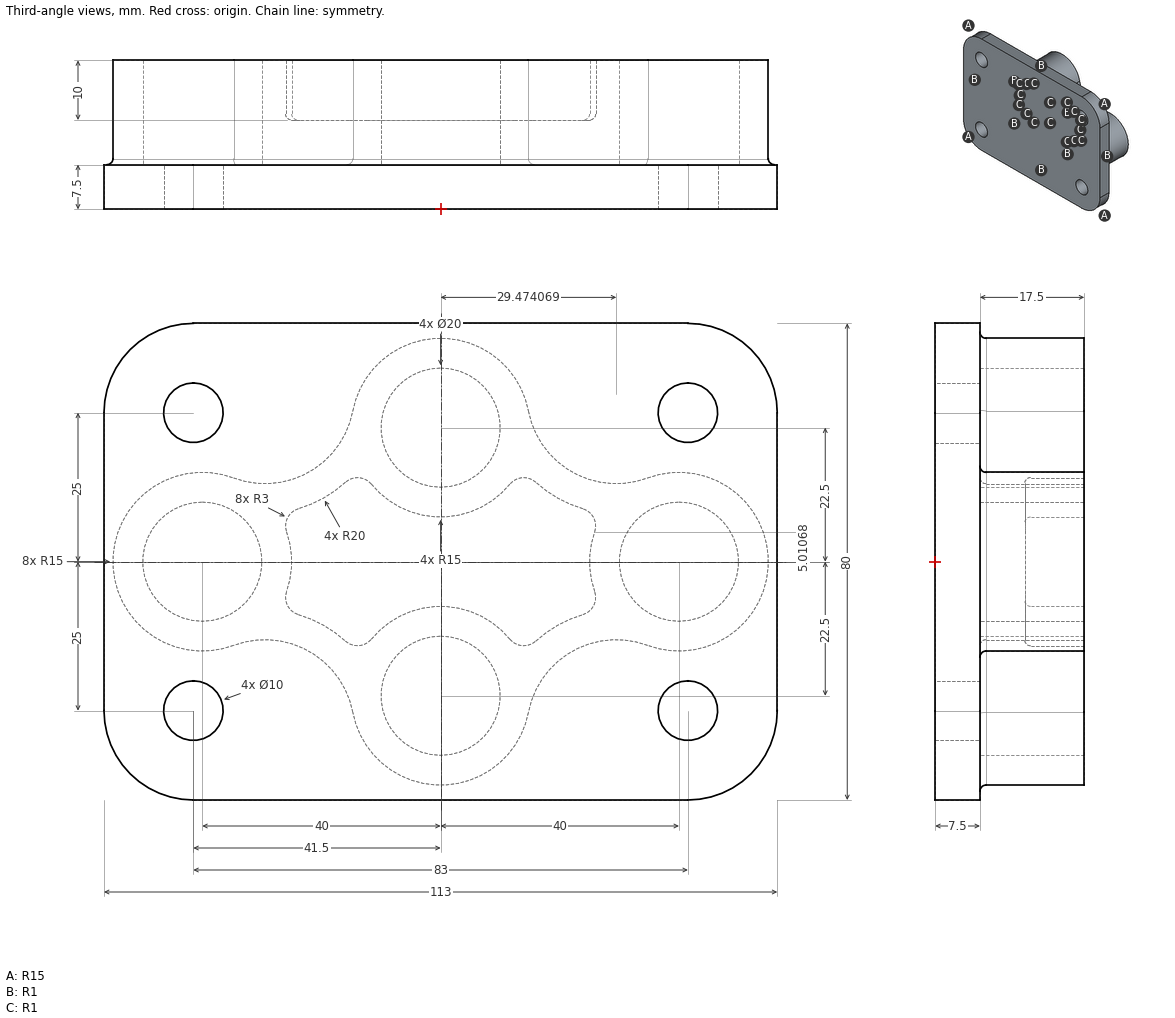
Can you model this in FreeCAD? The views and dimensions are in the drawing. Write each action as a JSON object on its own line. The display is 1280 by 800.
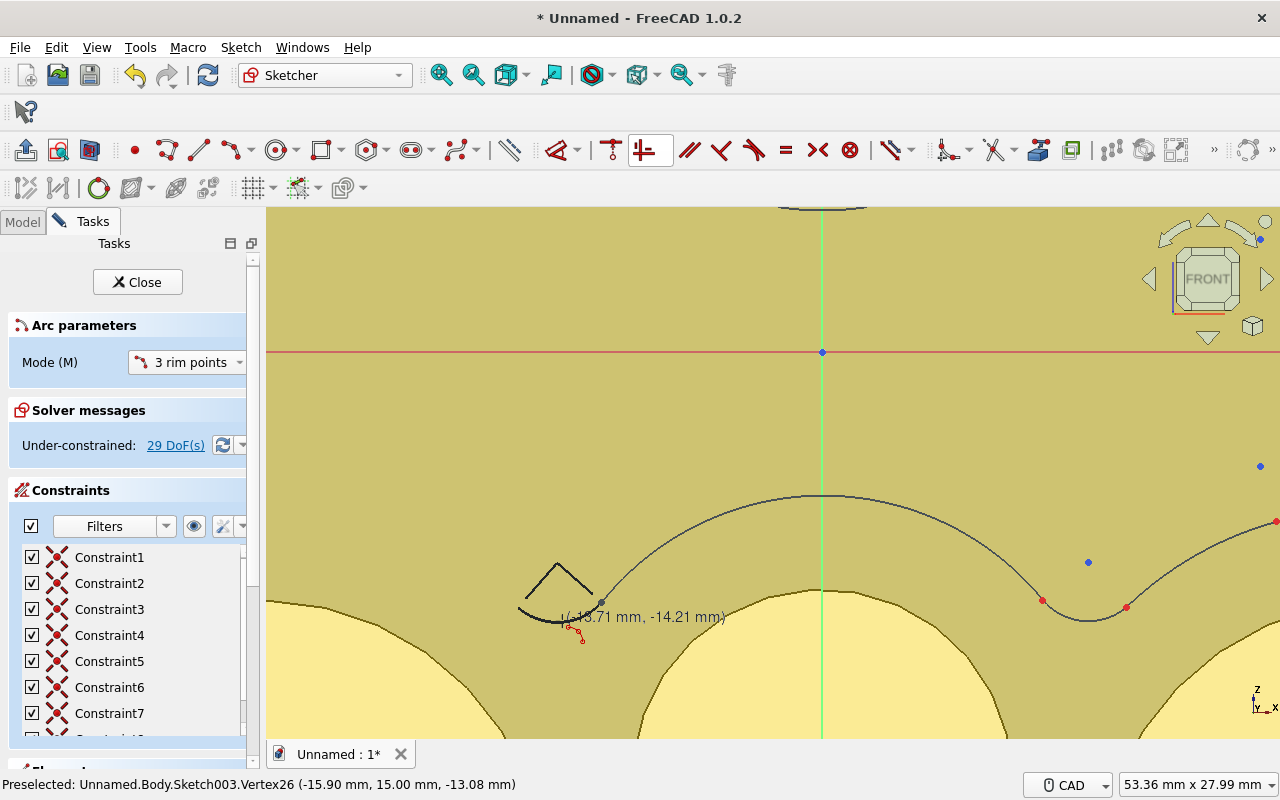
{"action": "left_click", "coordinate": [561, 620]}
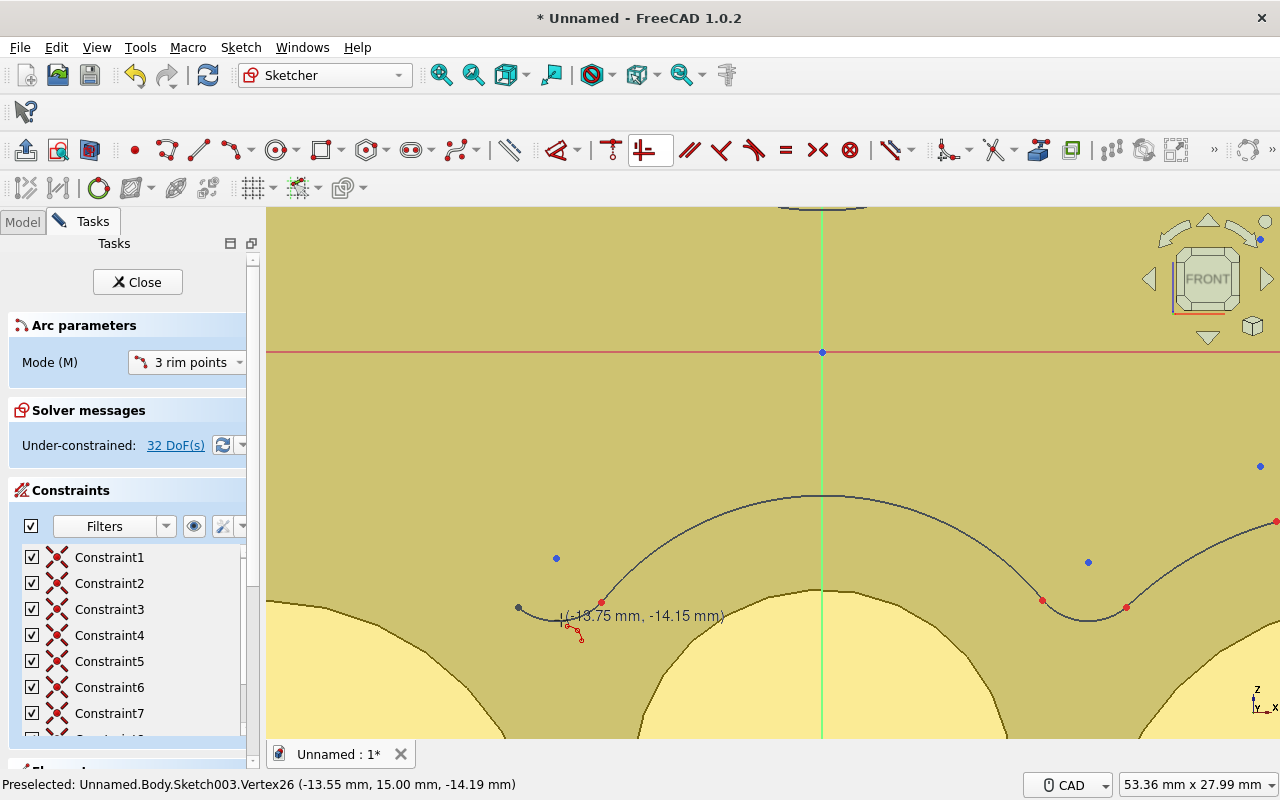
{"action": "left_click", "coordinate": [518, 608]}
{"action": "left_click", "coordinate": [369, 521]}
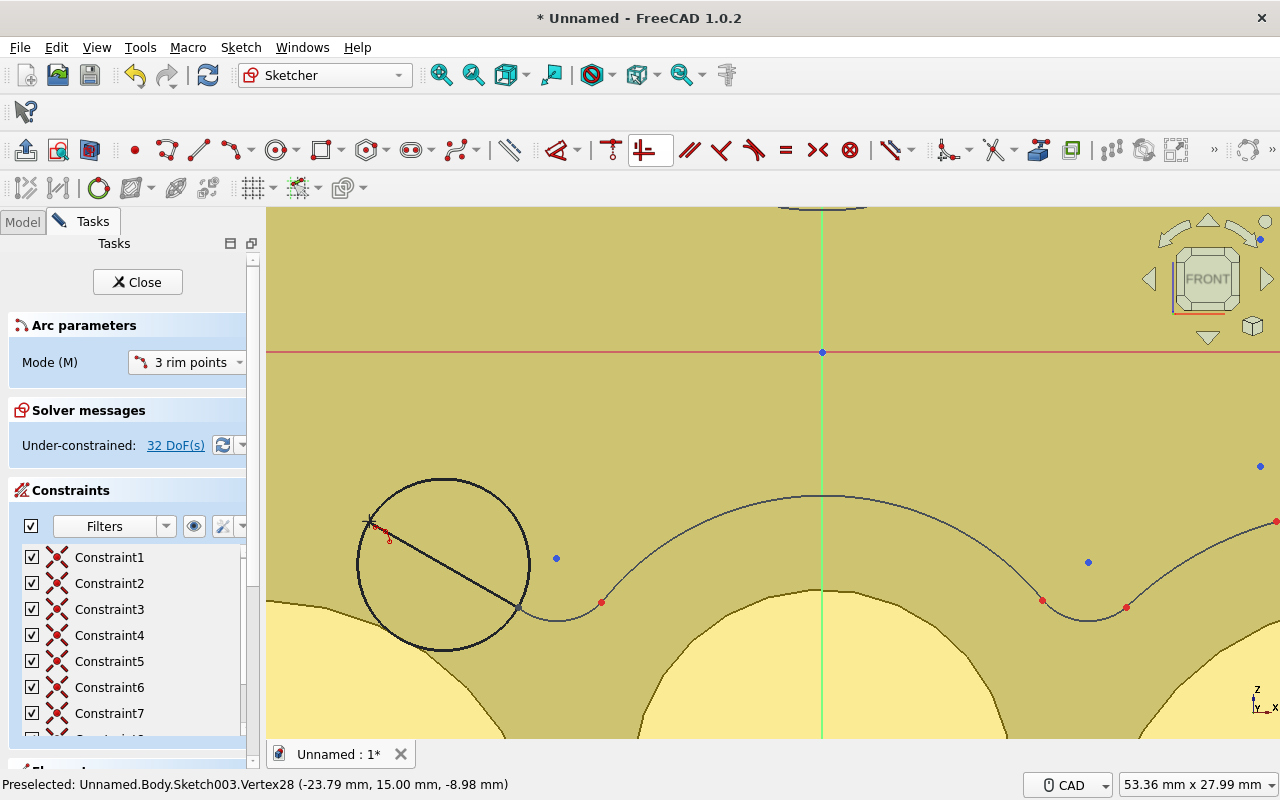
{"action": "scroll", "coordinate": [448, 555], "scroll_direction": "up", "scroll_amount": 3}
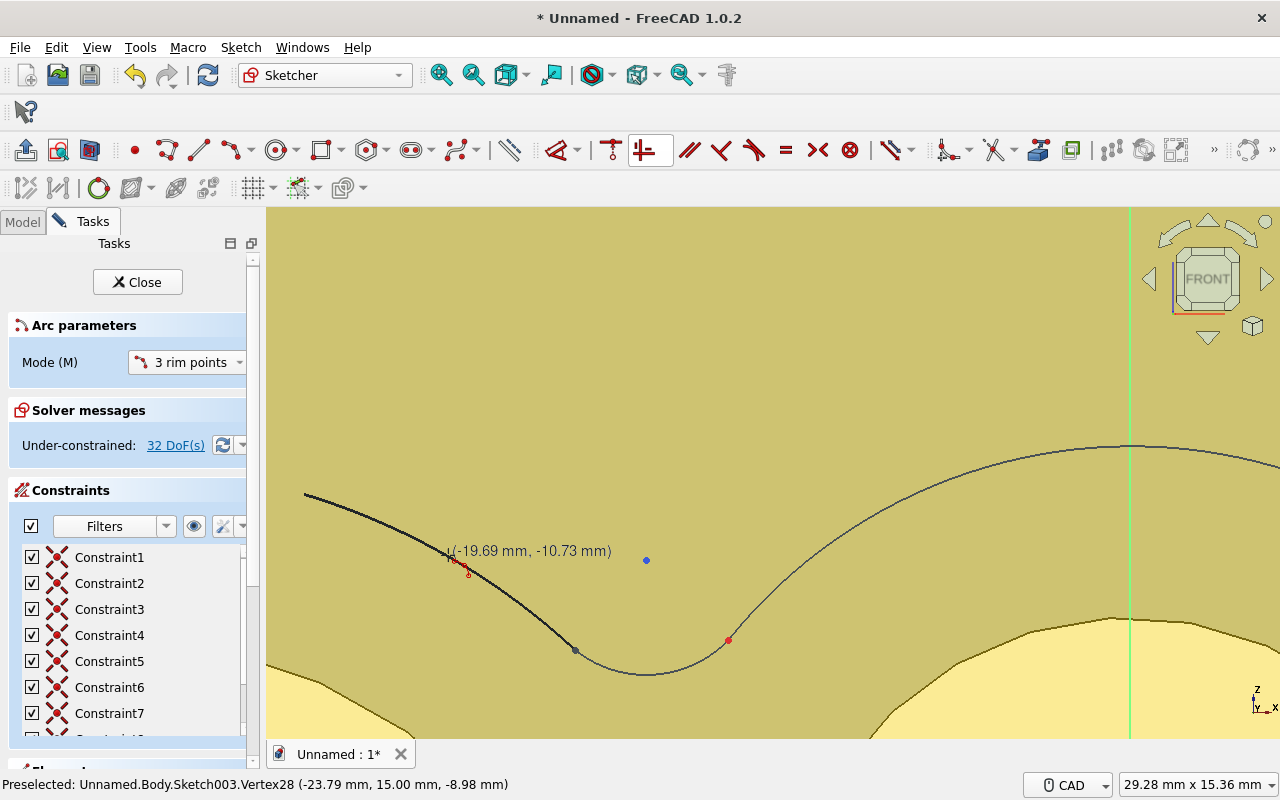
{"action": "left_click", "coordinate": [449, 554]}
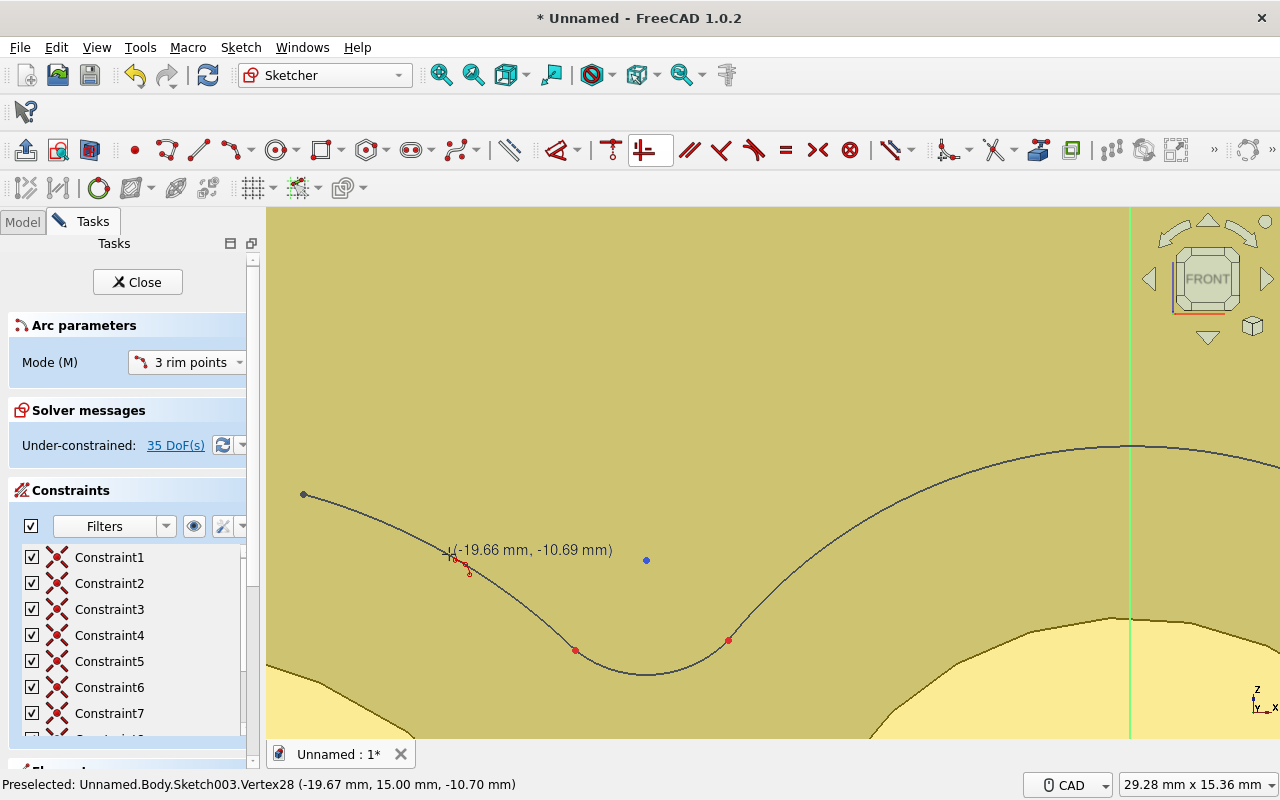
{"action": "left_click", "coordinate": [304, 494]}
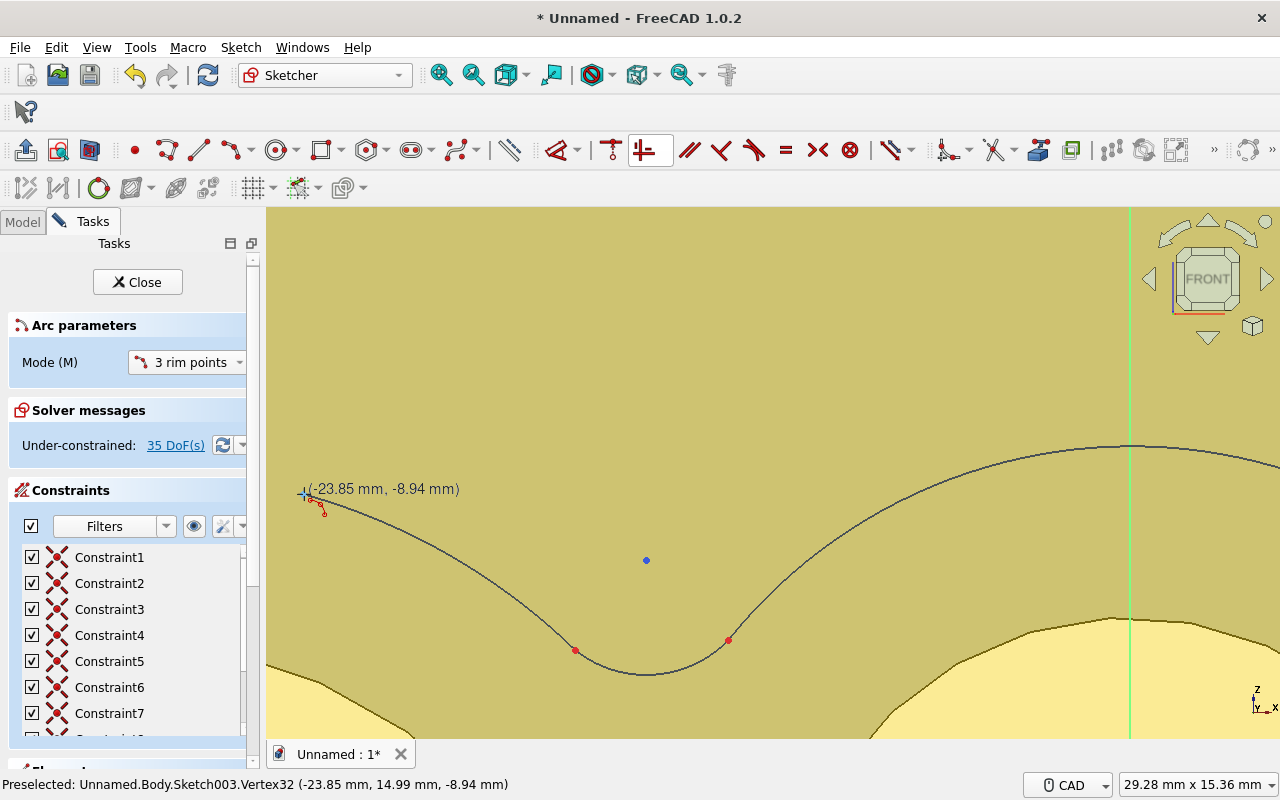
{"action": "scroll", "coordinate": [521, 597], "scroll_direction": "down", "scroll_amount": 6}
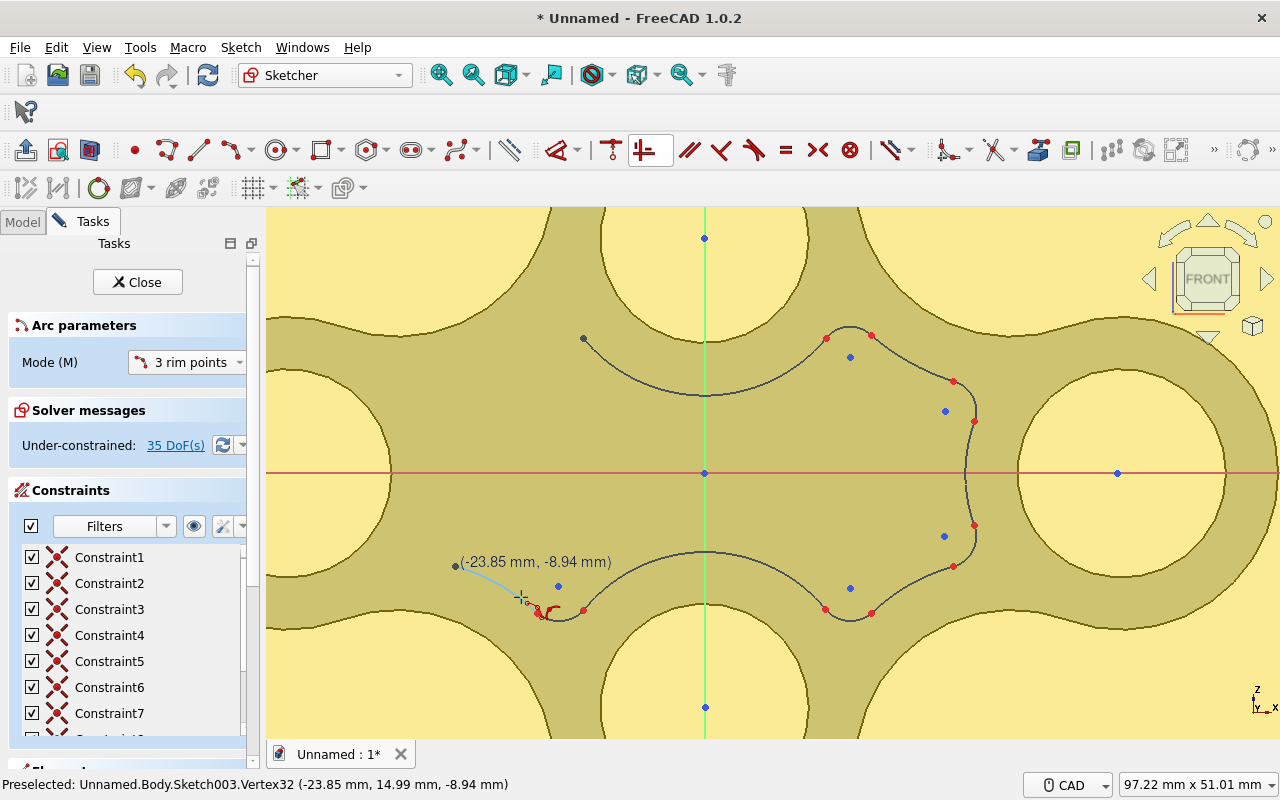
{"action": "left_click", "coordinate": [435, 526]}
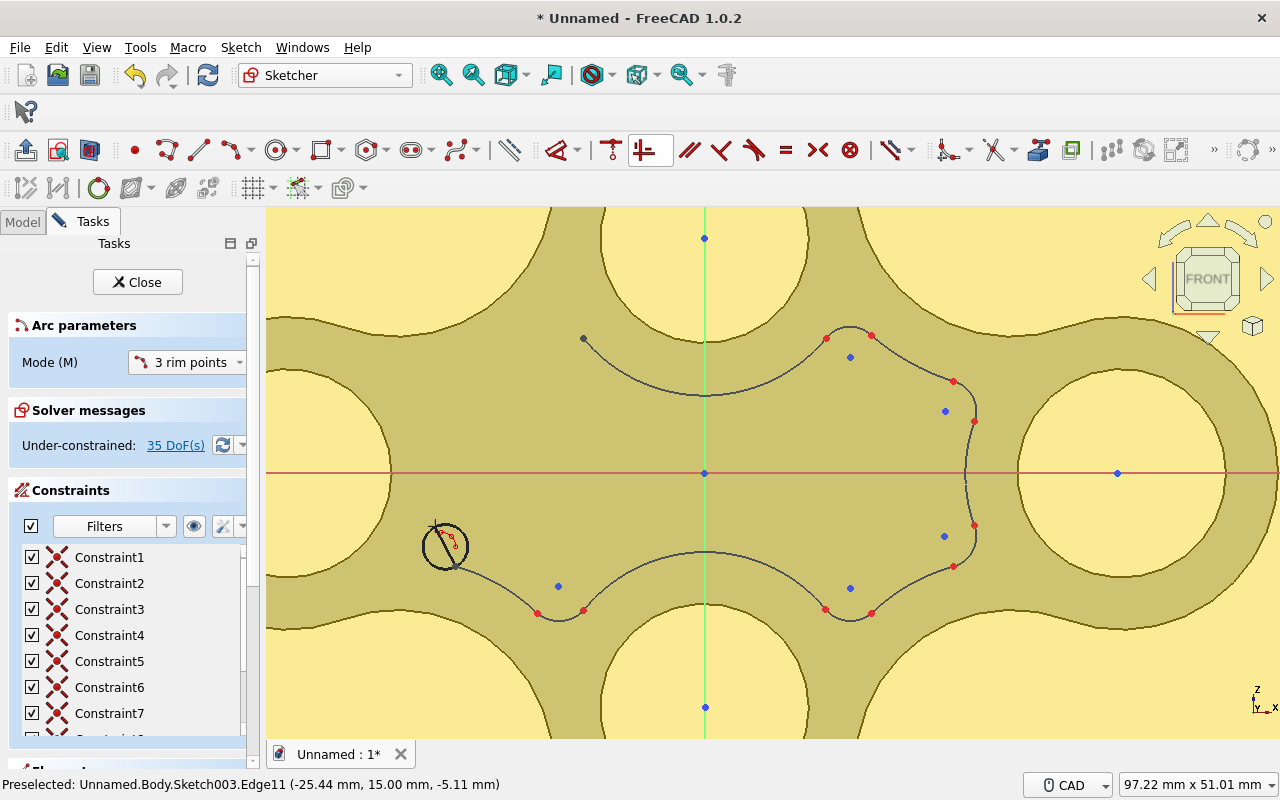
{"action": "scroll", "coordinate": [436, 550], "scroll_direction": "up", "scroll_amount": 3}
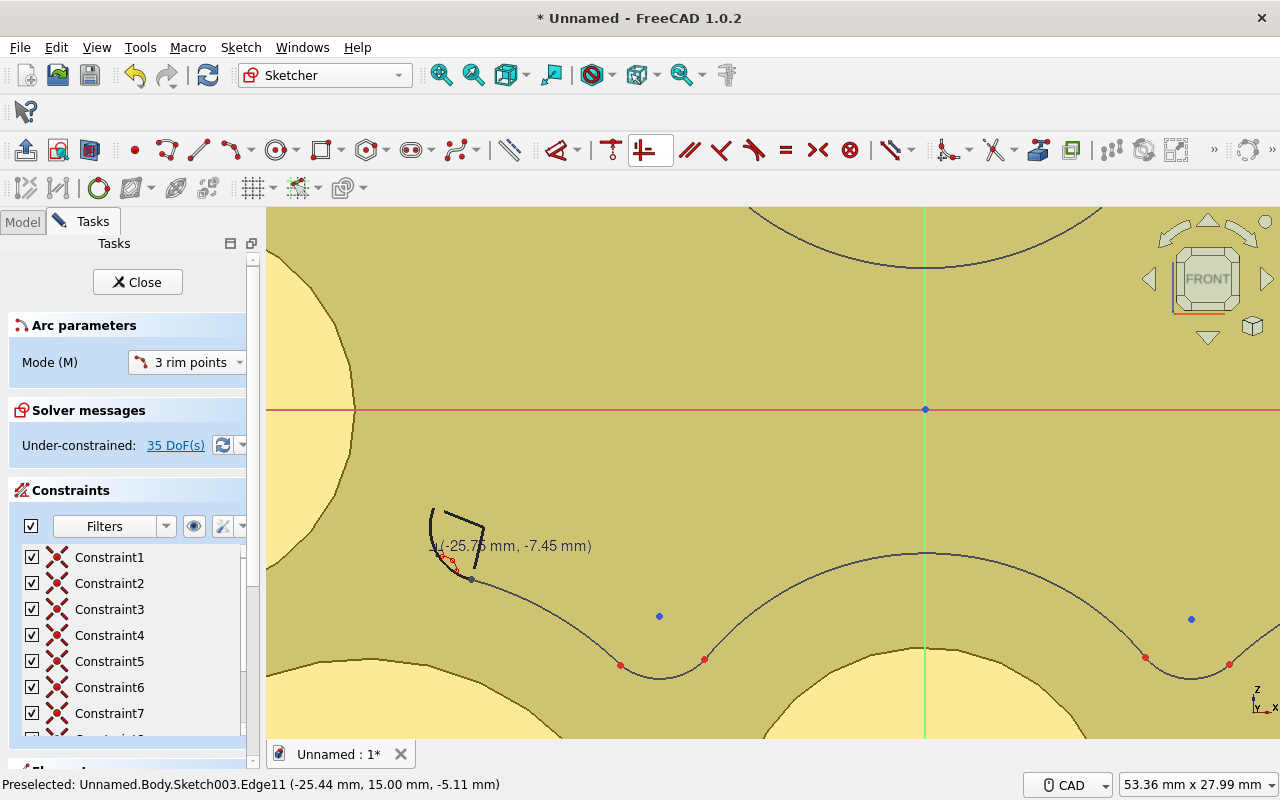
{"action": "left_click", "coordinate": [437, 550]}